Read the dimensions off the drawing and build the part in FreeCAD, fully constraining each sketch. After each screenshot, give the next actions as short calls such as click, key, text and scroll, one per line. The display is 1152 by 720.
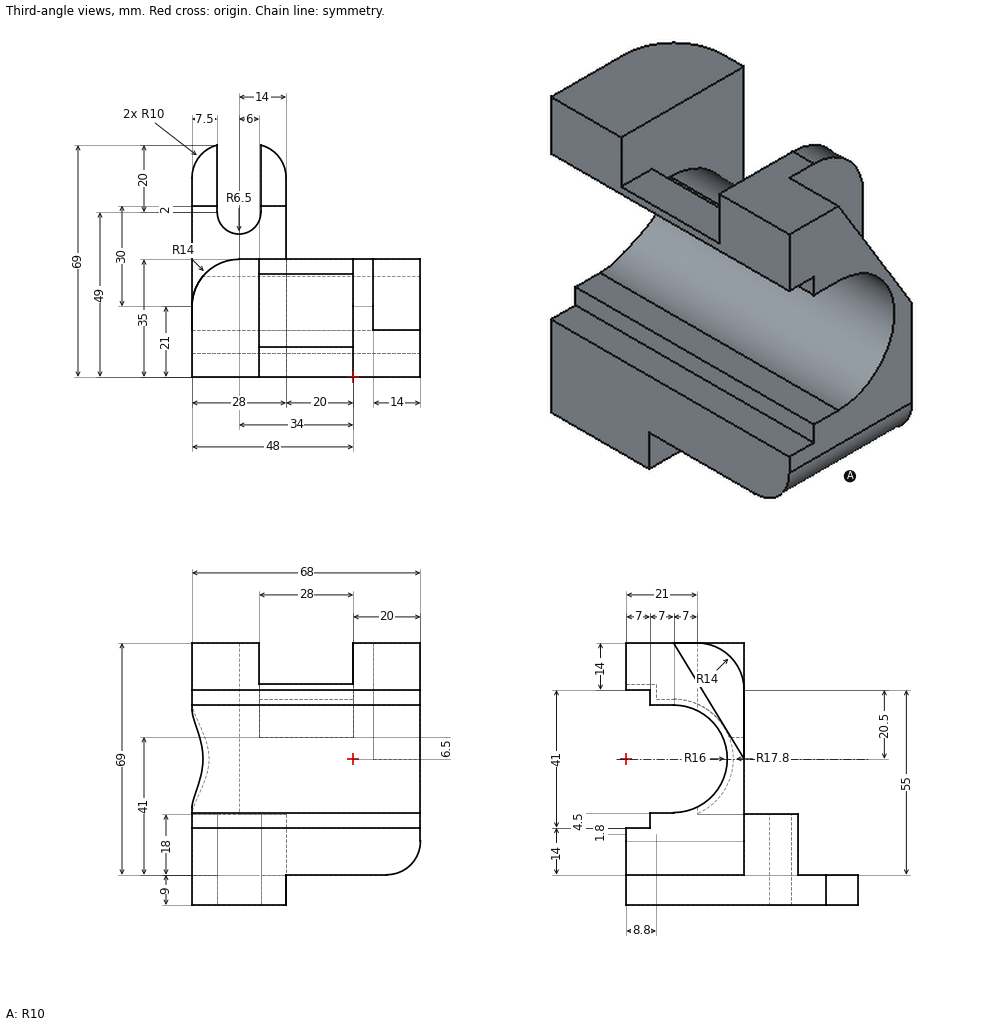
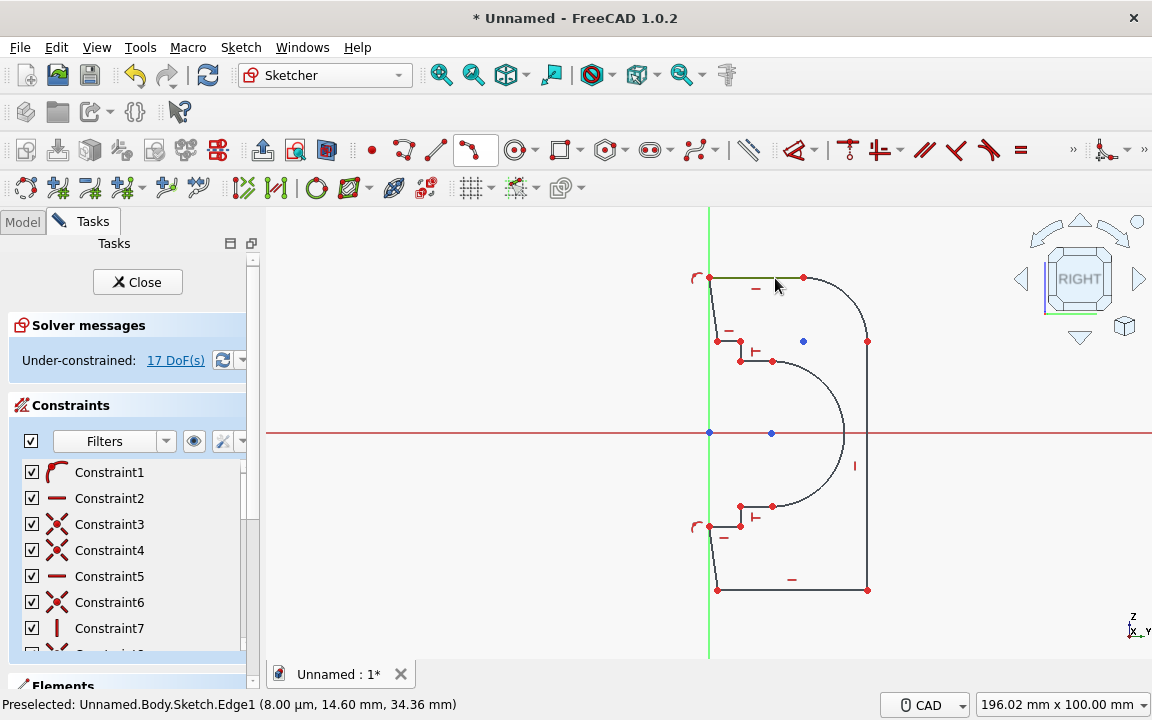
click(860, 313)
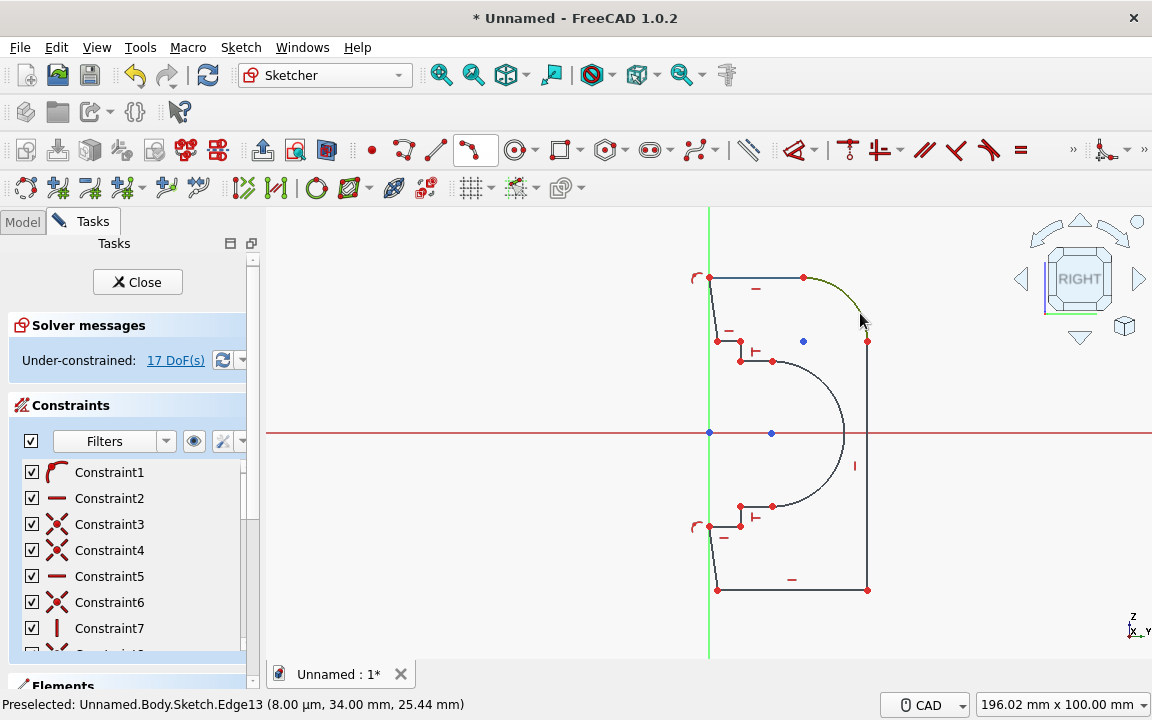
click(990, 150)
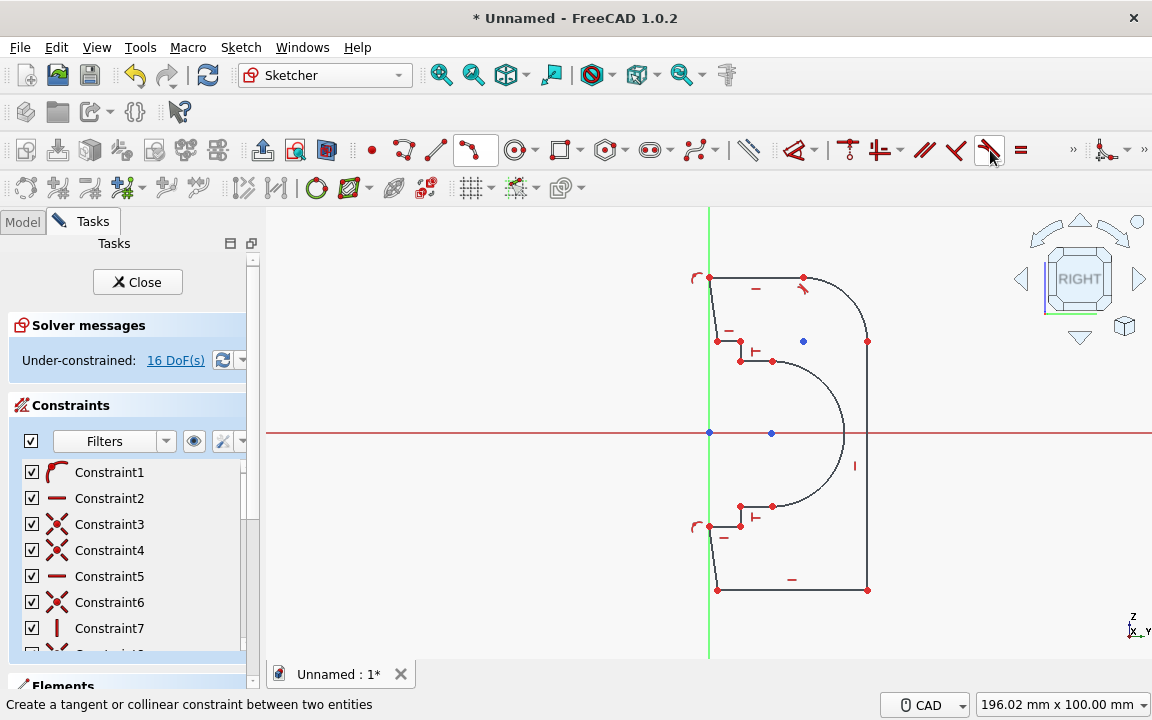
scroll(750, 361, up, 2)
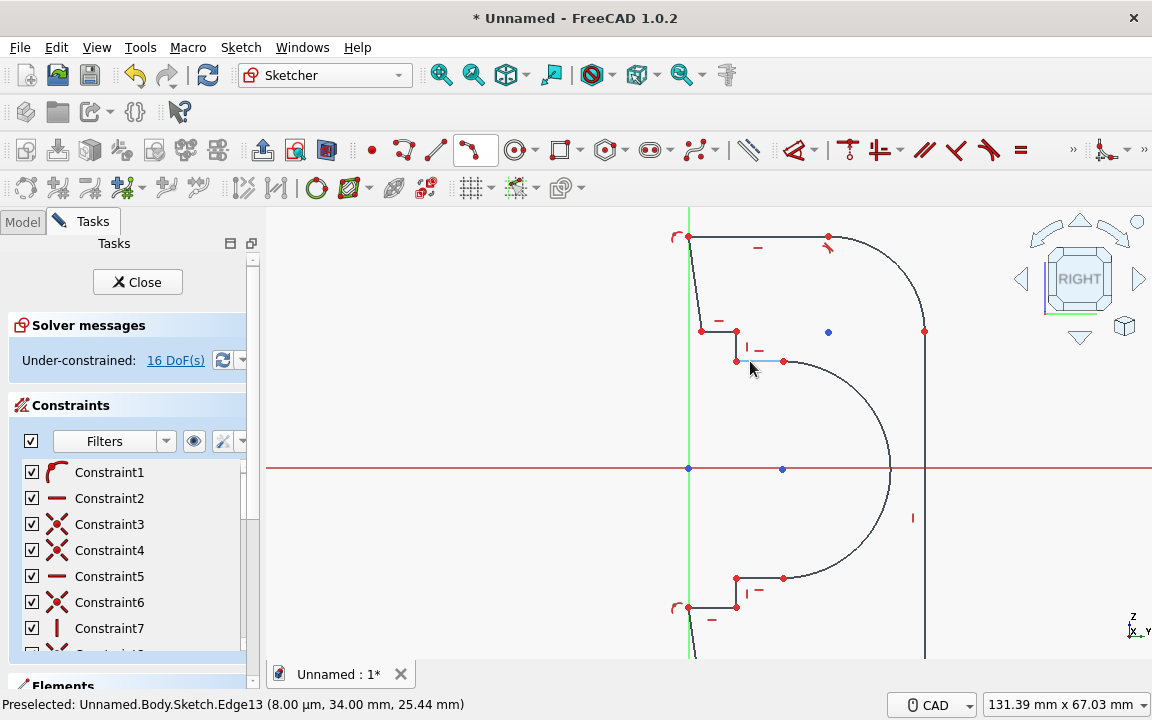
click(750, 361)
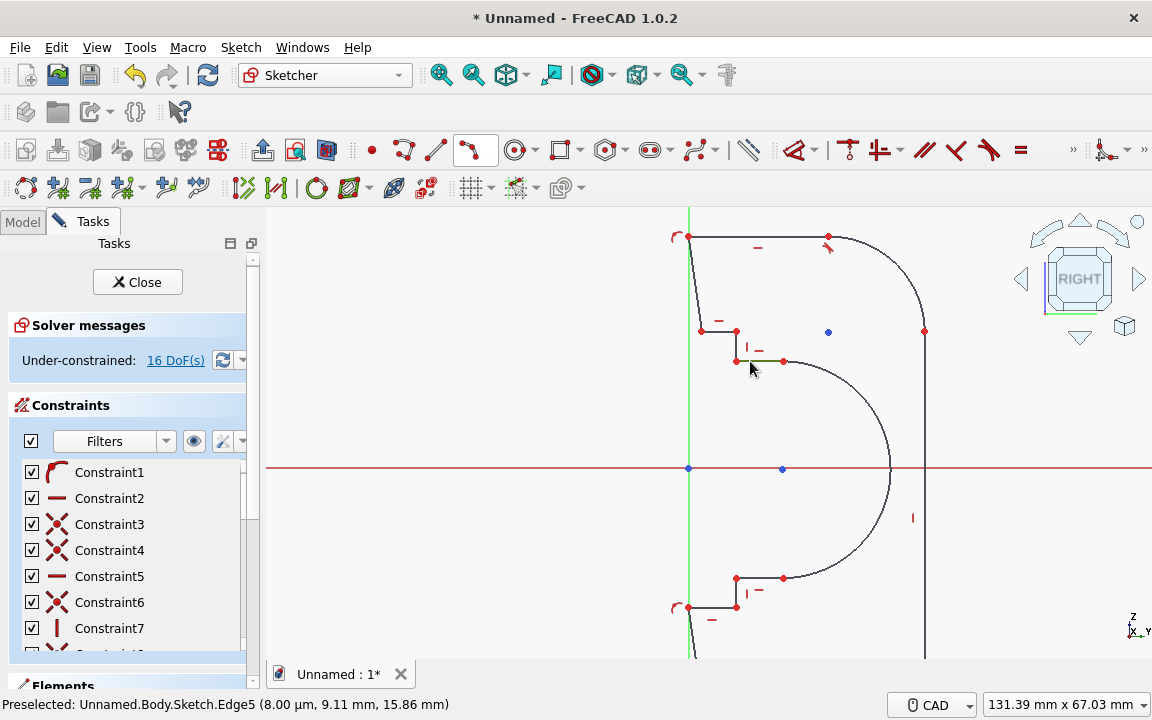
click(870, 533)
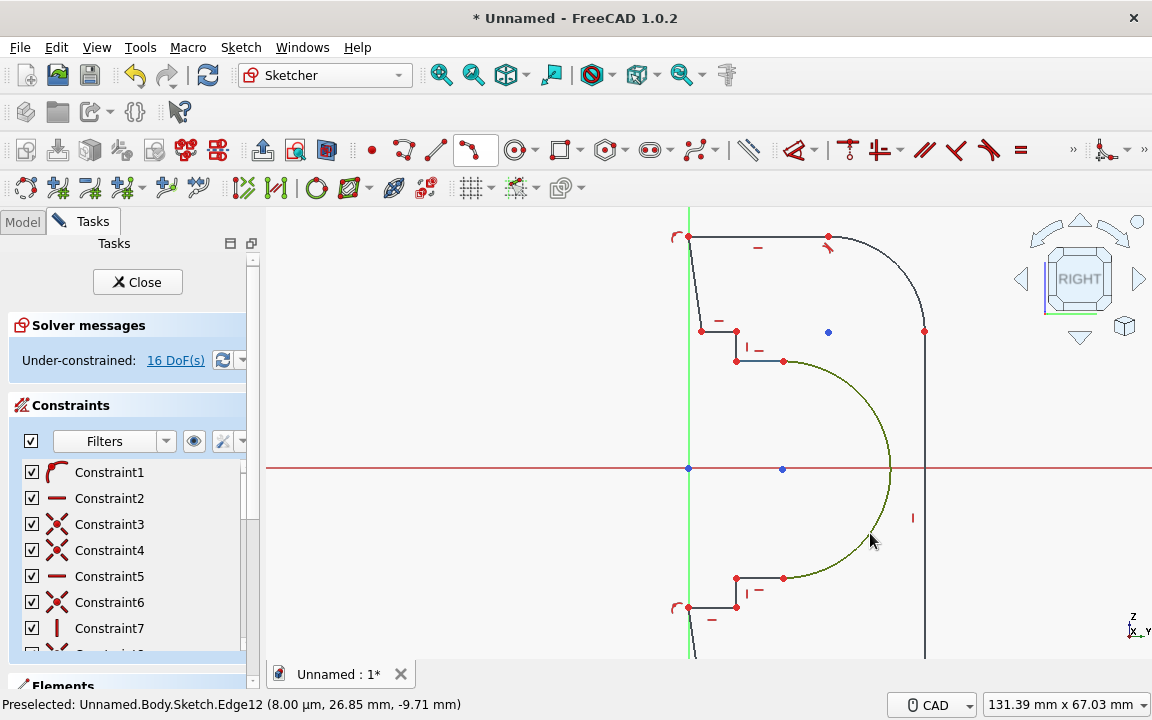
click(990, 150)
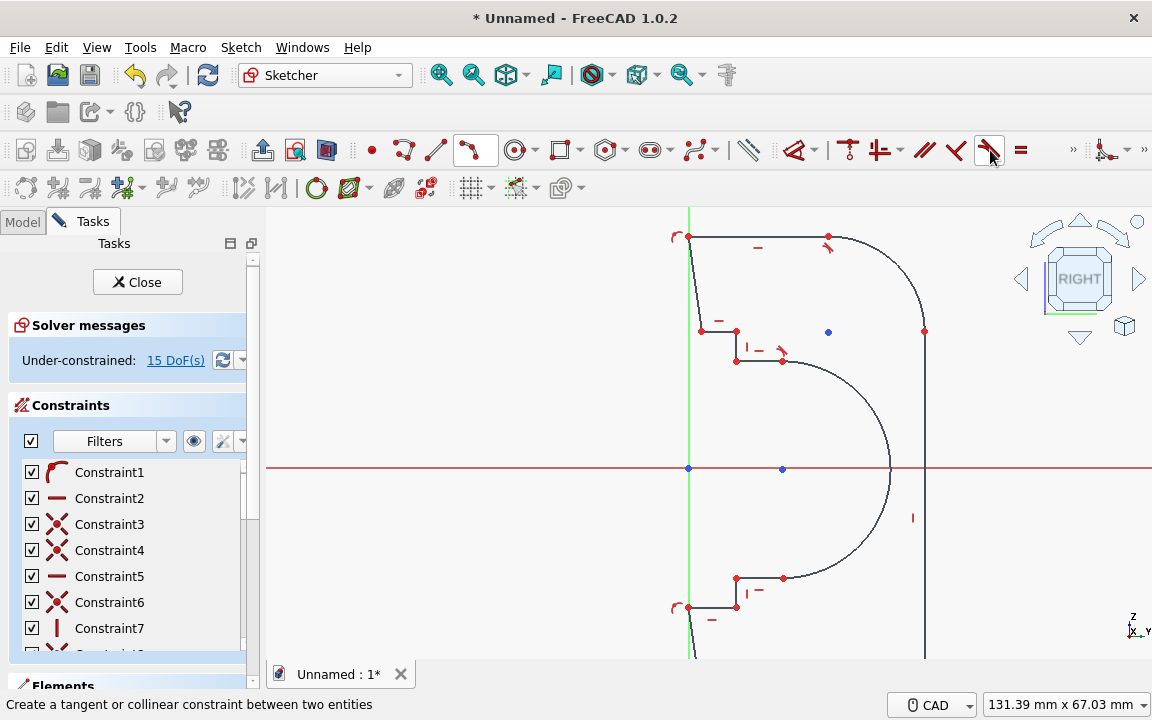
click(769, 578)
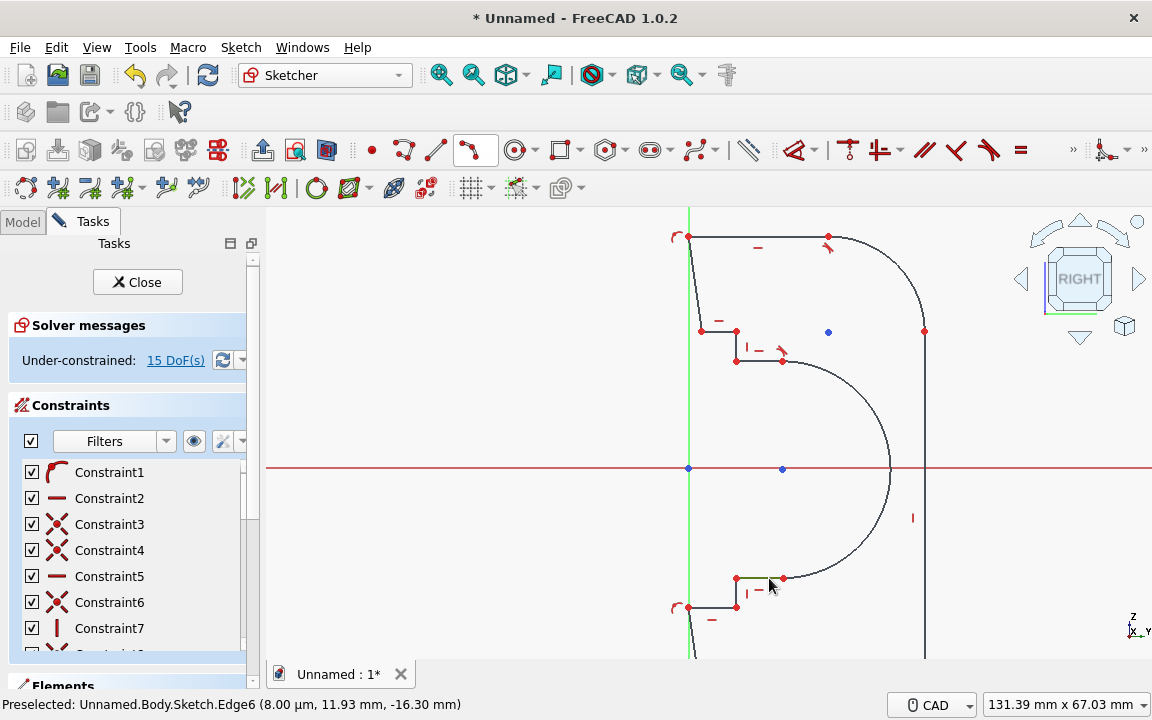
click(870, 533)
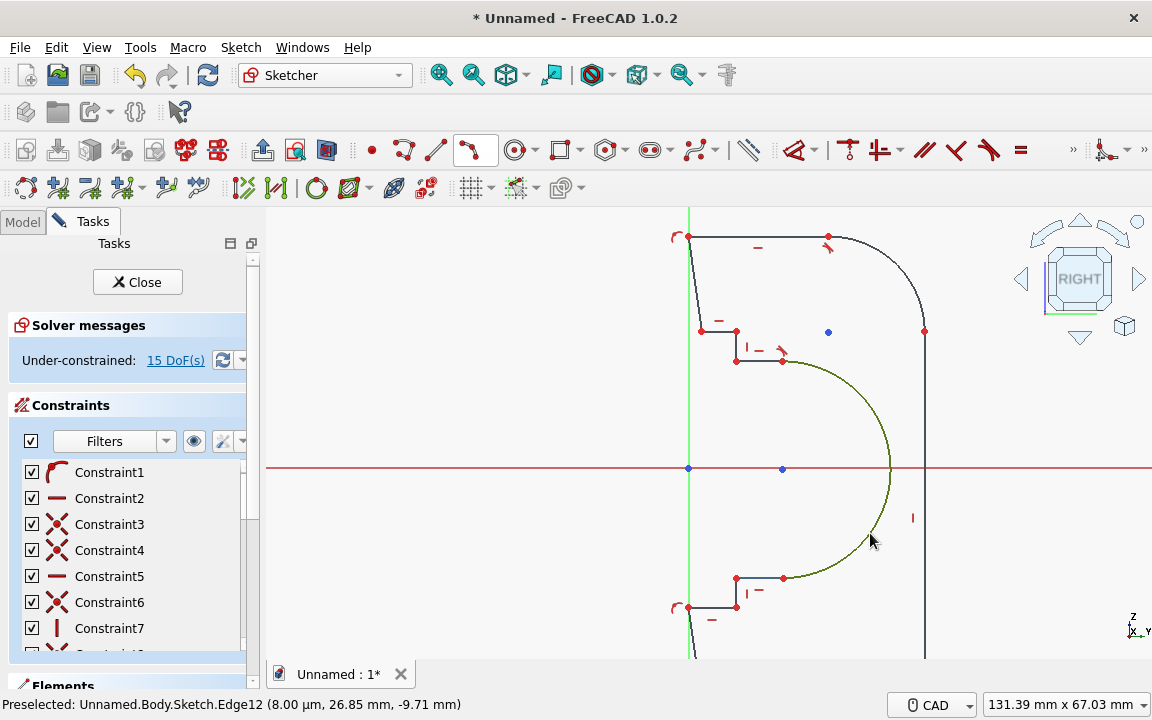
click(990, 150)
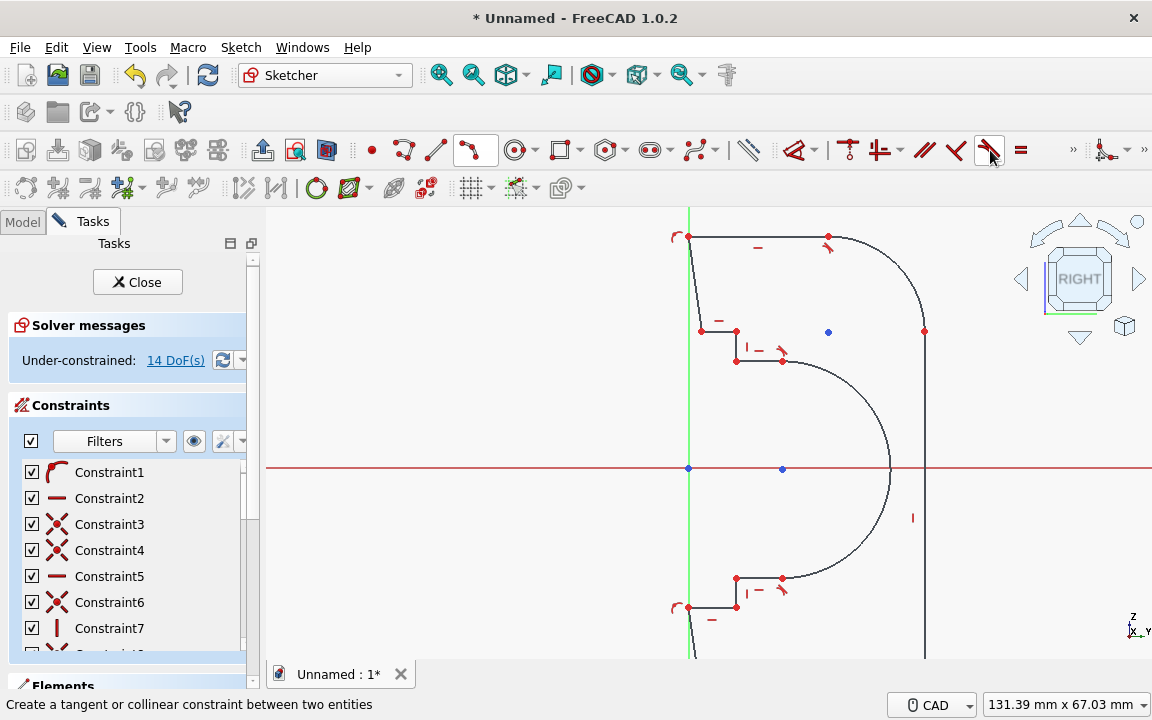
click(925, 592)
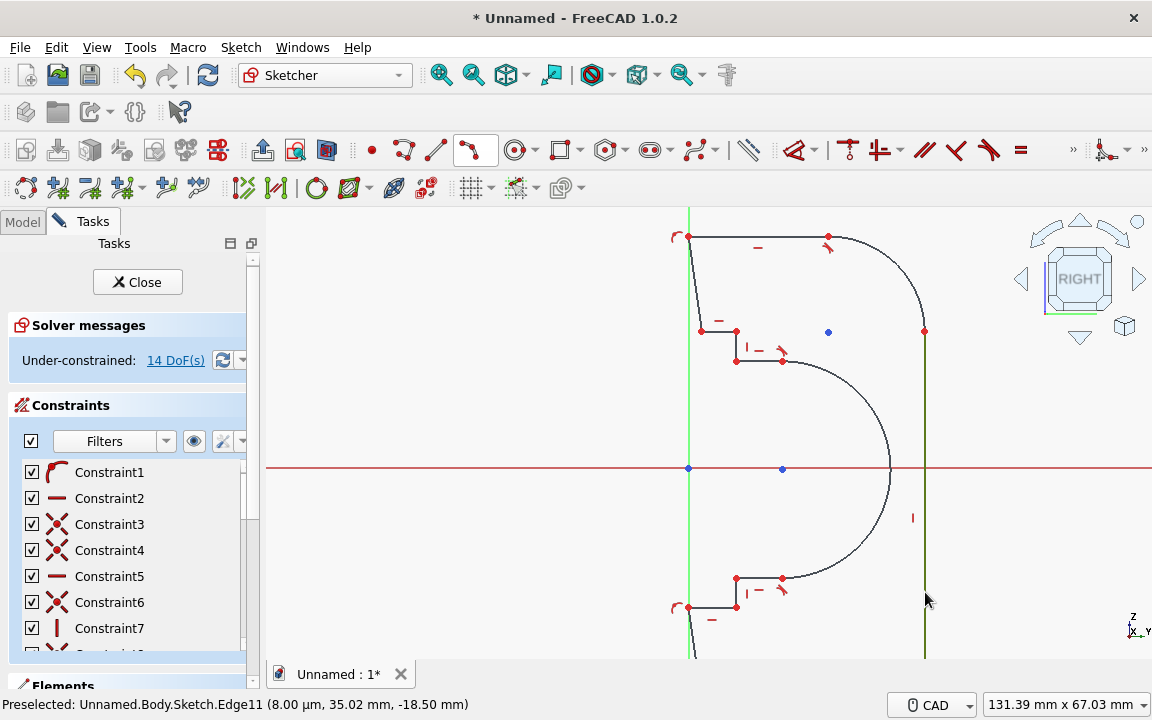
click(914, 288)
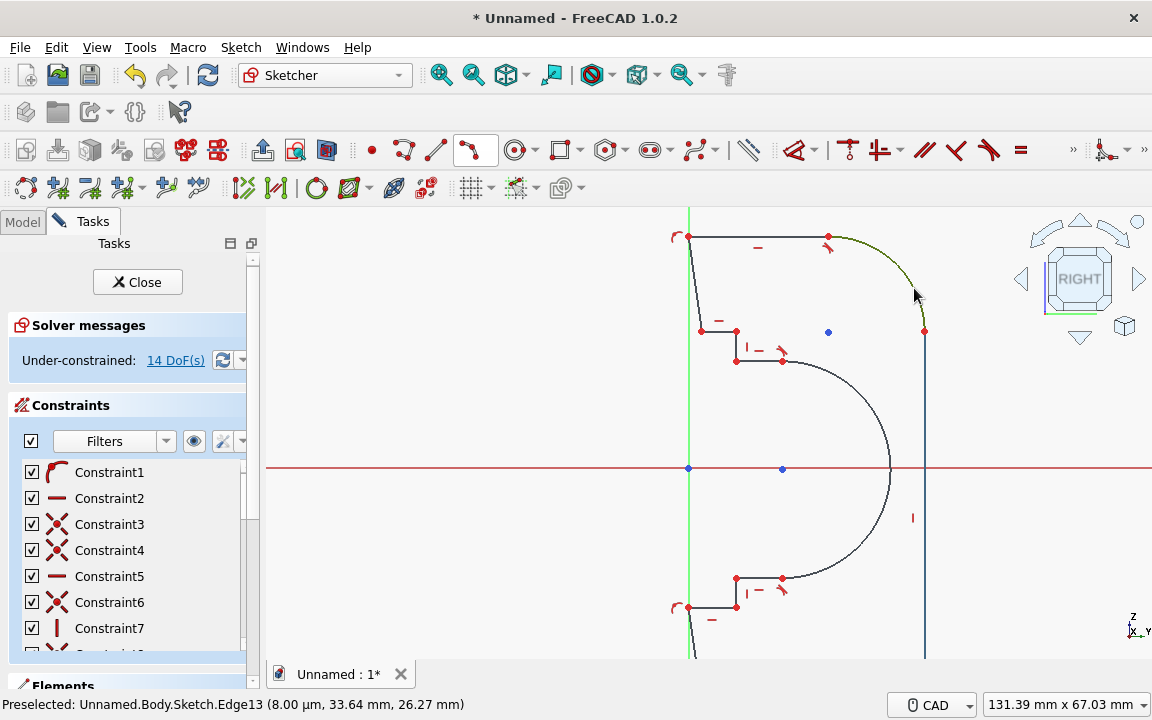
click(990, 150)